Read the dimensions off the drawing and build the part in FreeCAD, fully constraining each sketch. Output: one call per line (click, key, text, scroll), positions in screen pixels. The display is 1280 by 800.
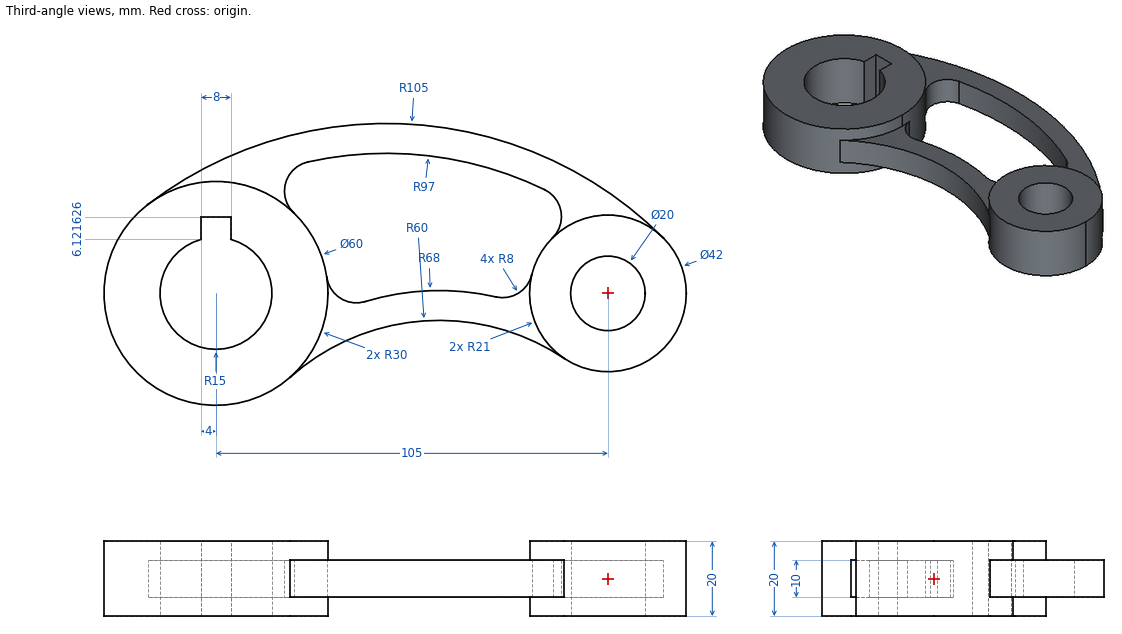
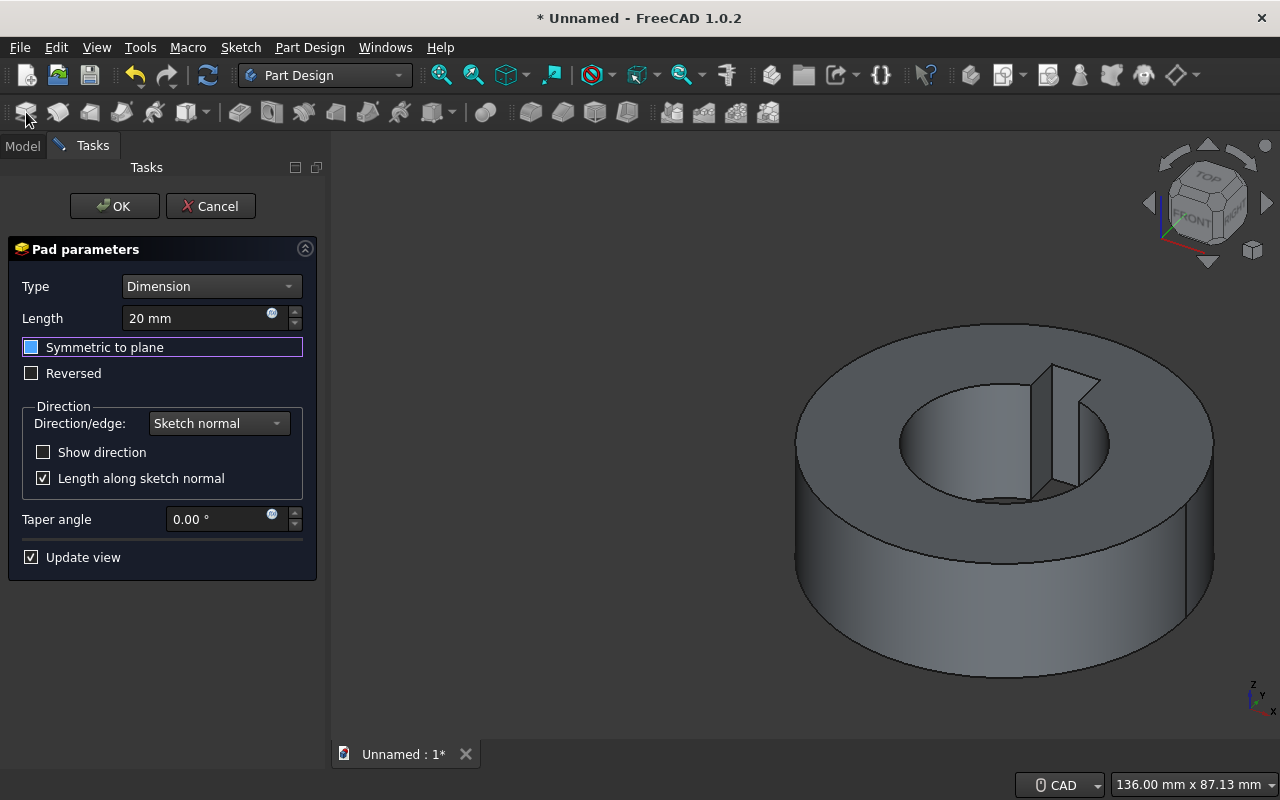
click(30, 347)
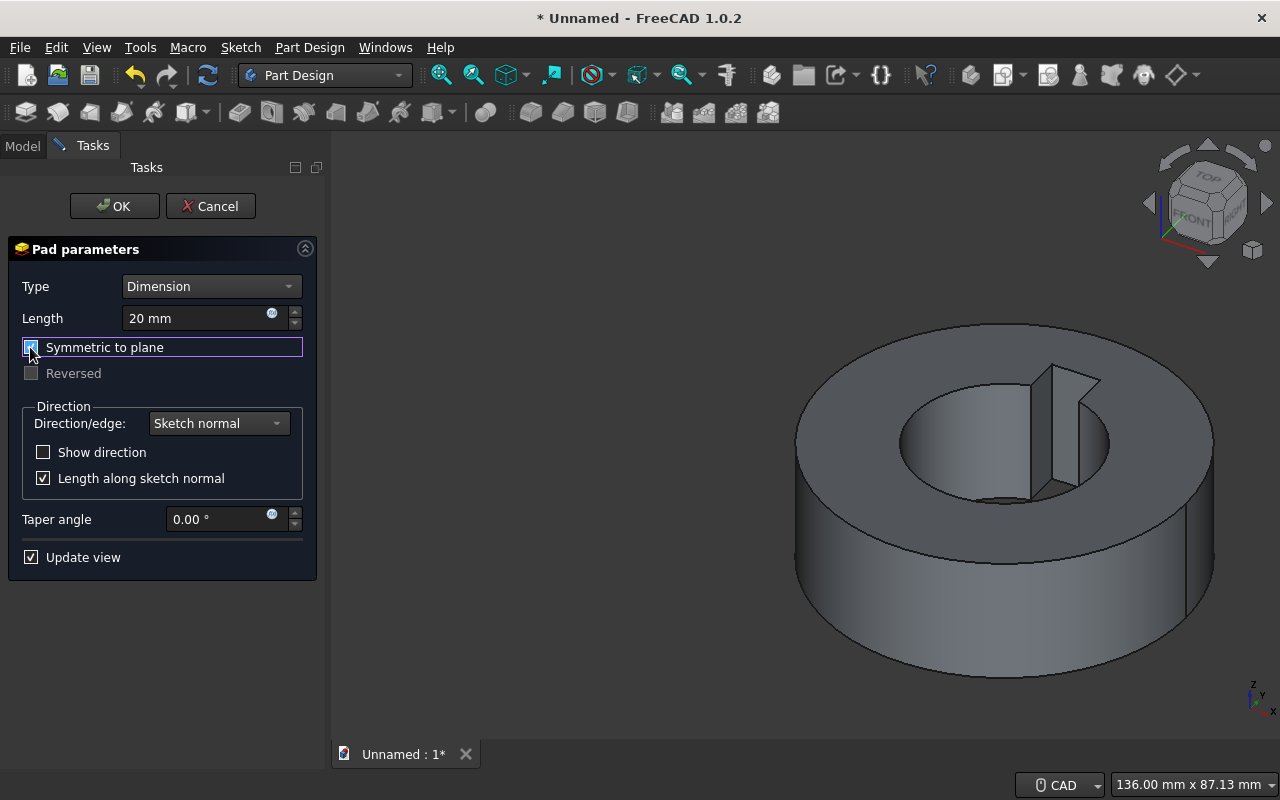
click(115, 206)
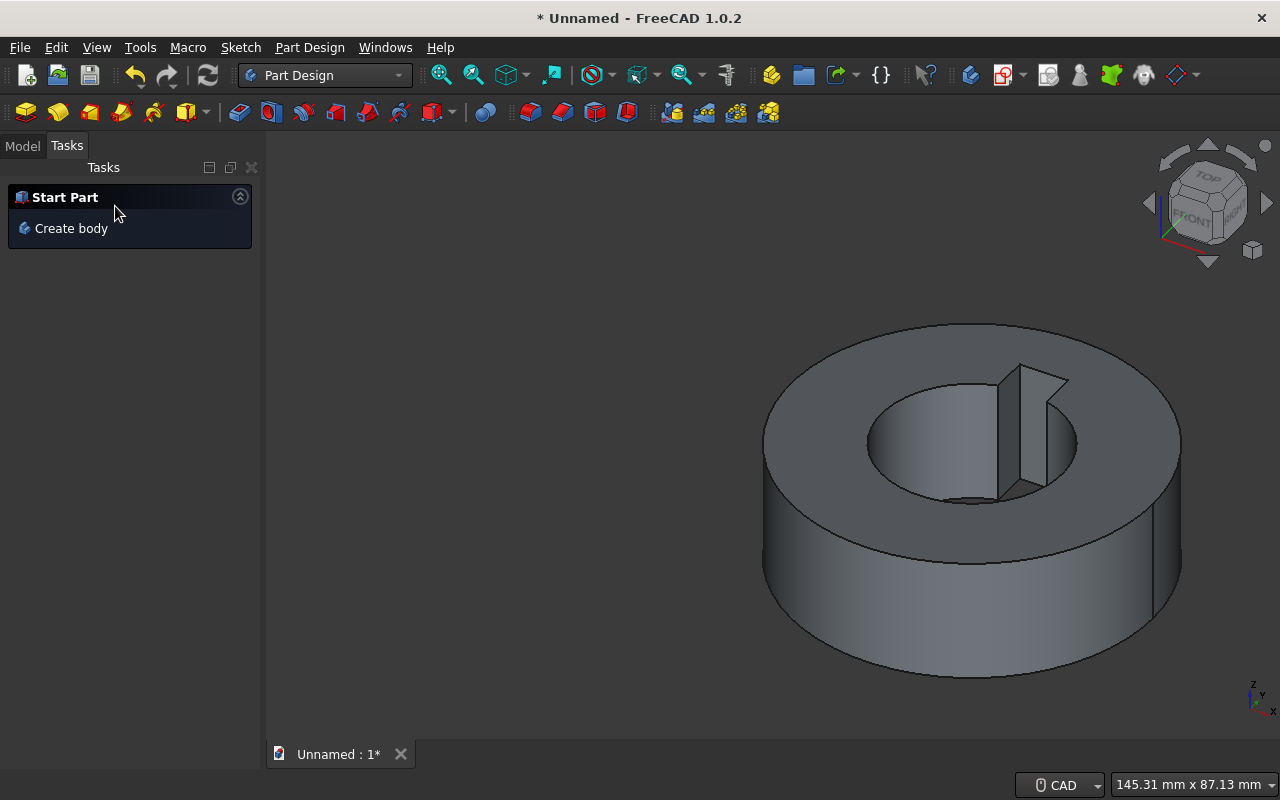
click(442, 76)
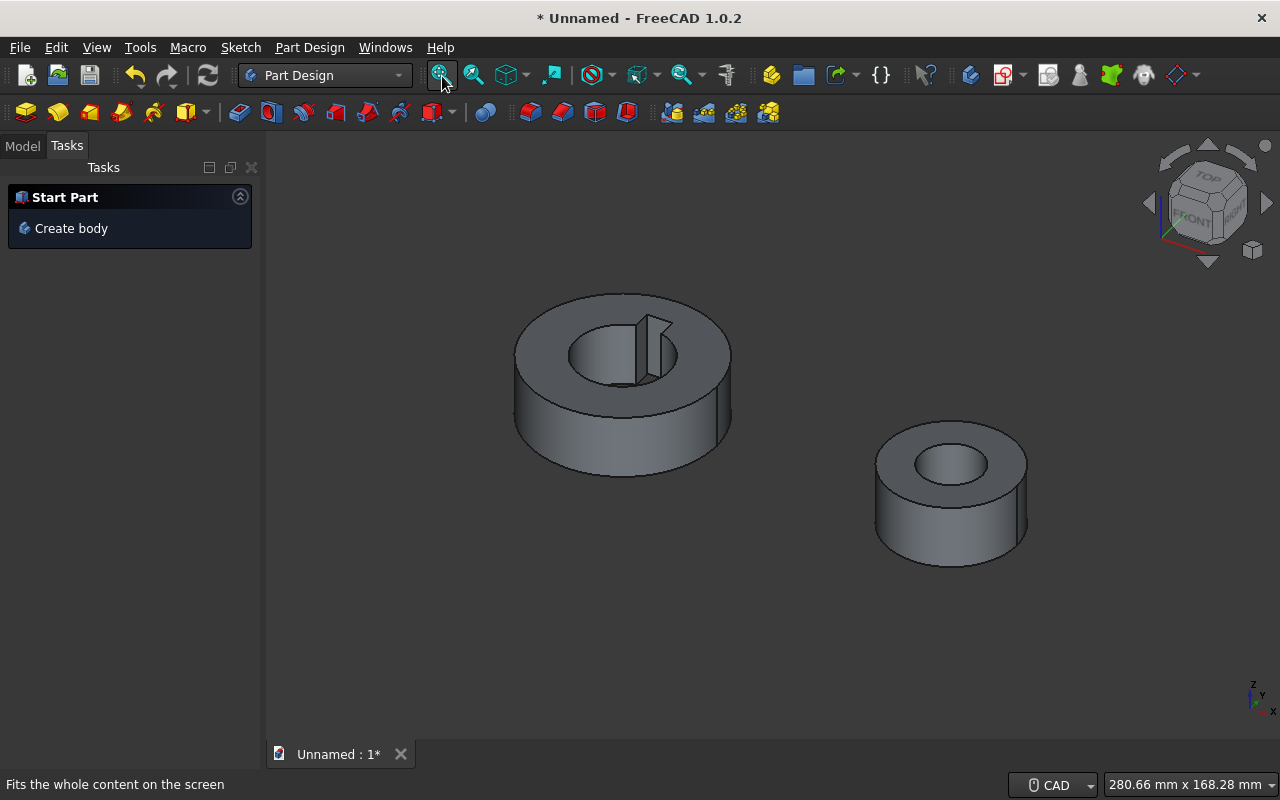
click(23, 145)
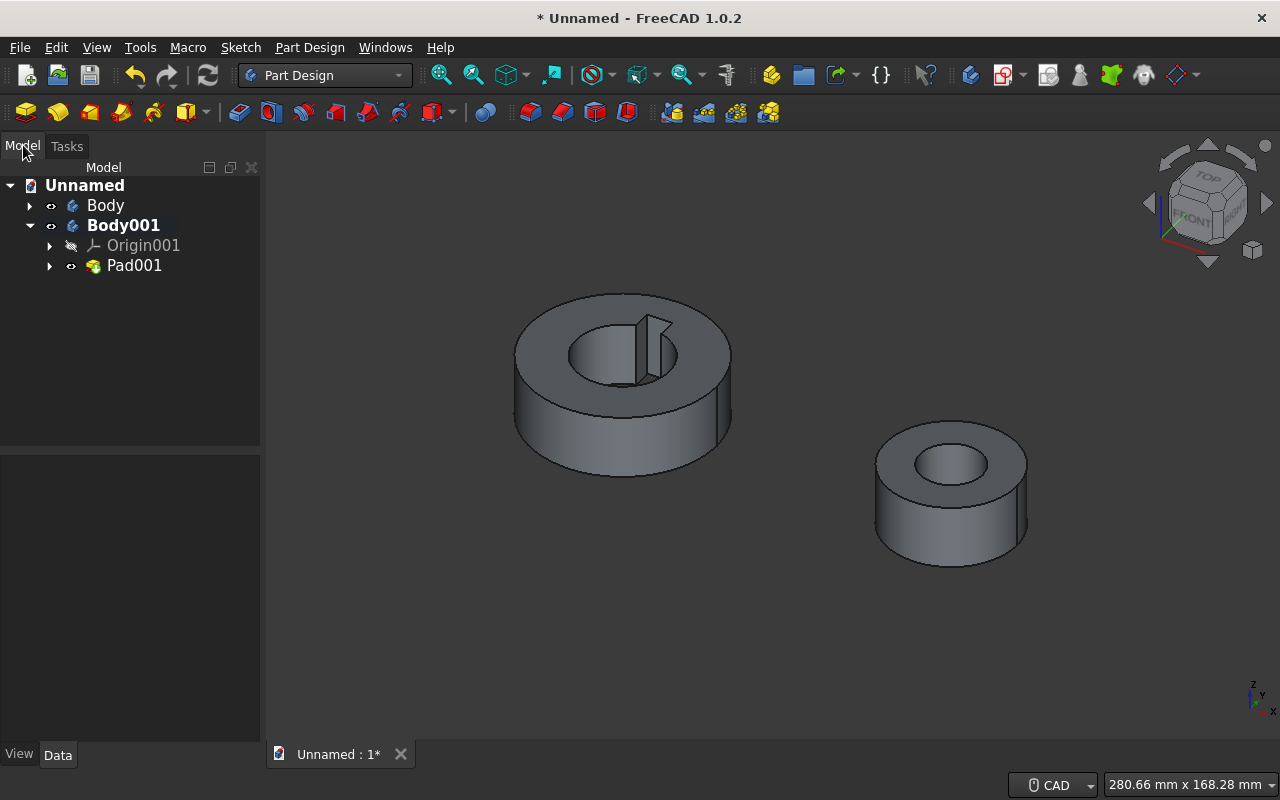
double_click(96, 206)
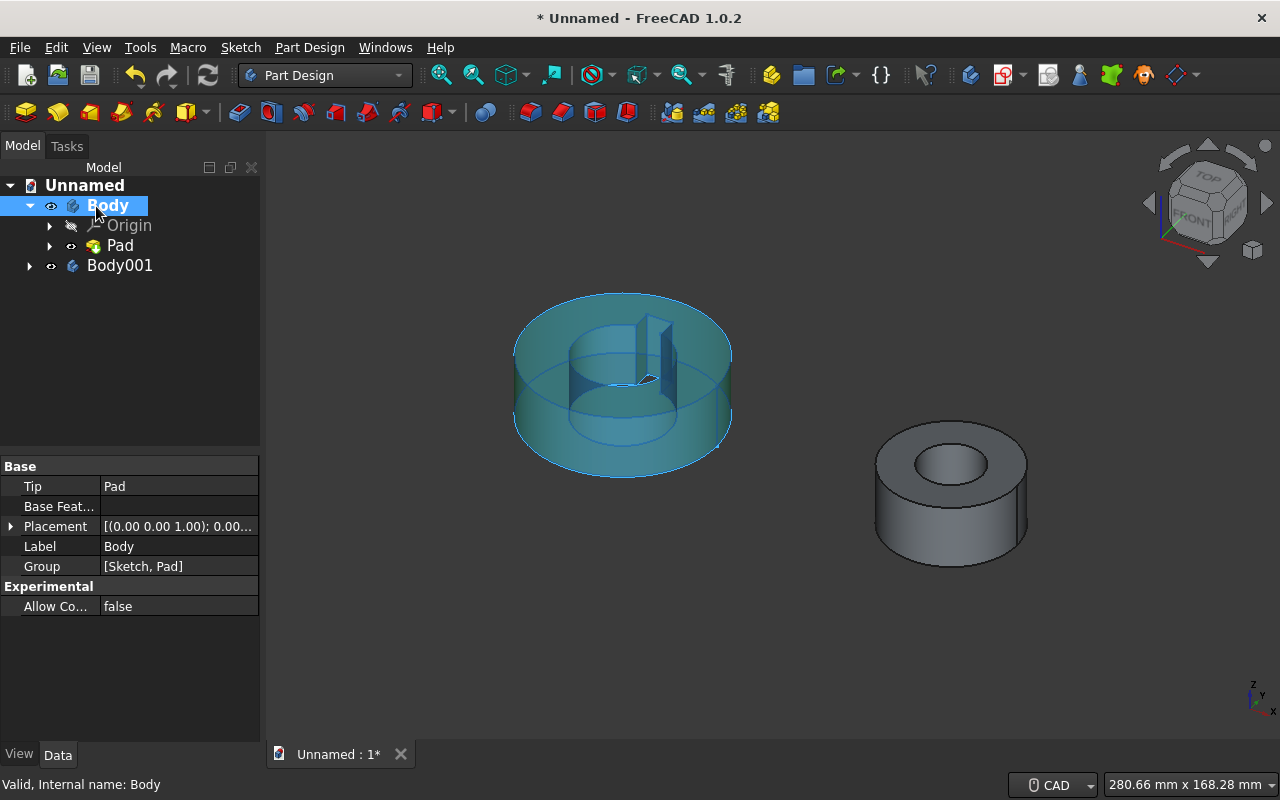
click(96, 206)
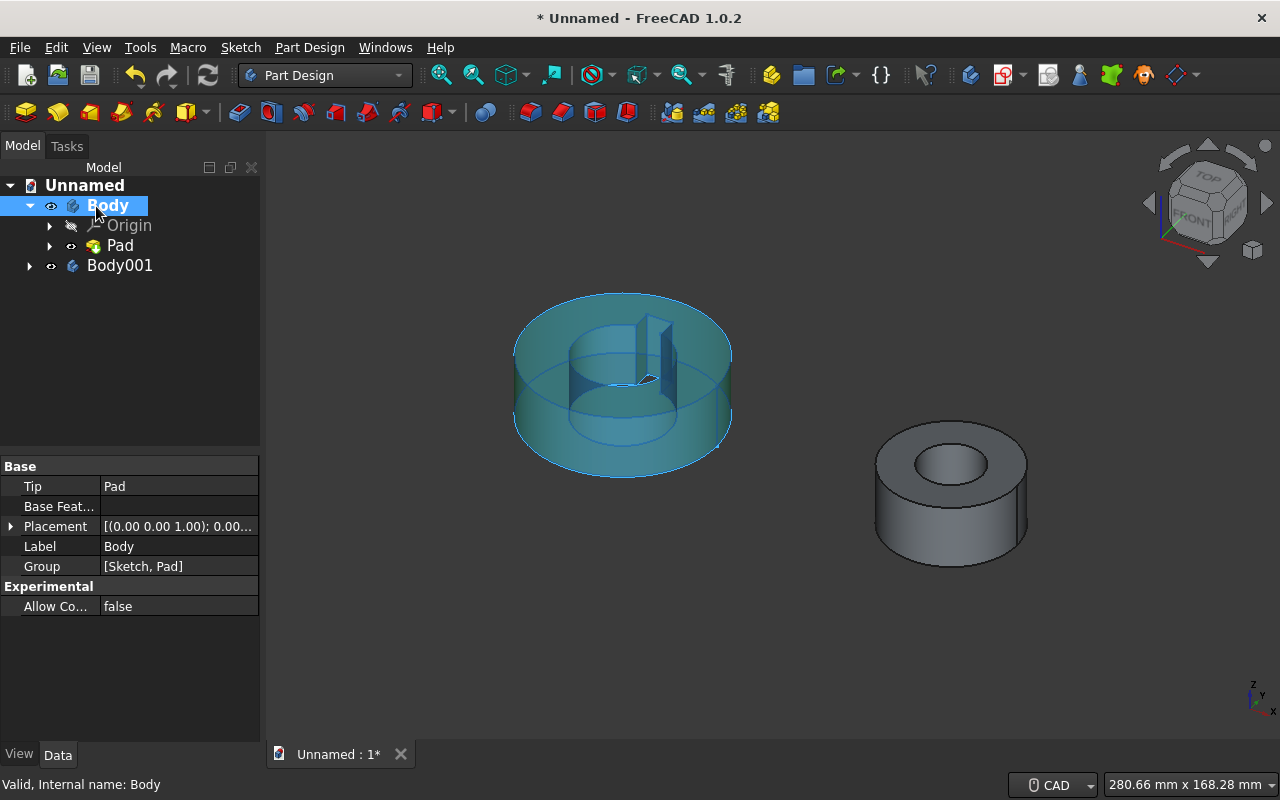
click(146, 606)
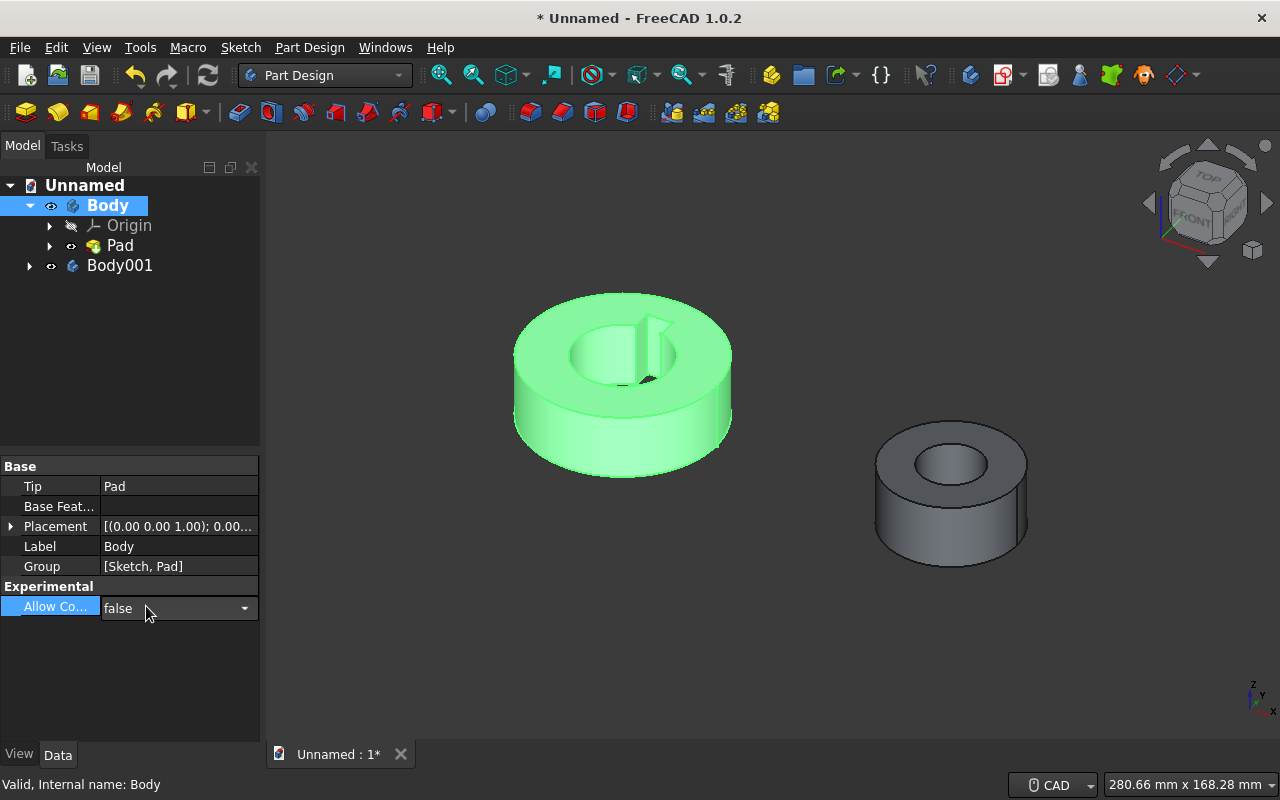
click(146, 606)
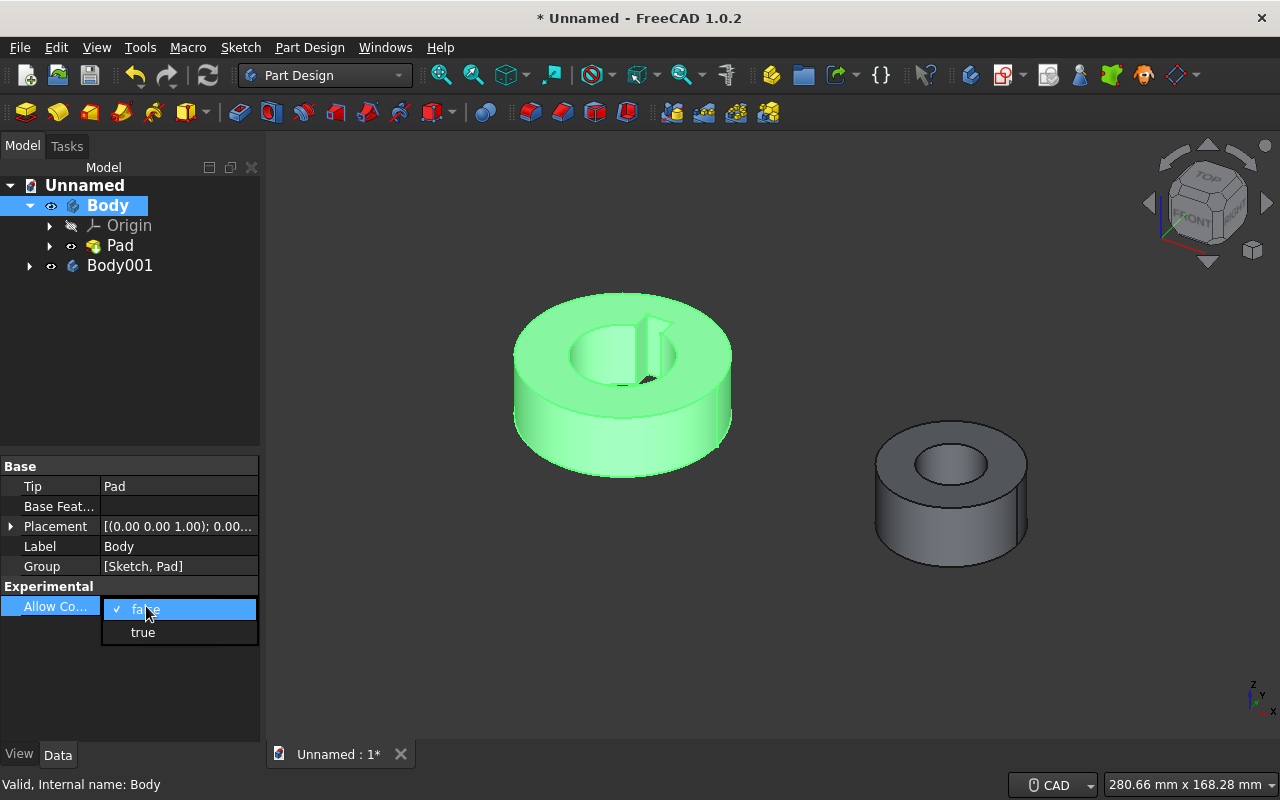
click(179, 632)
key(Return)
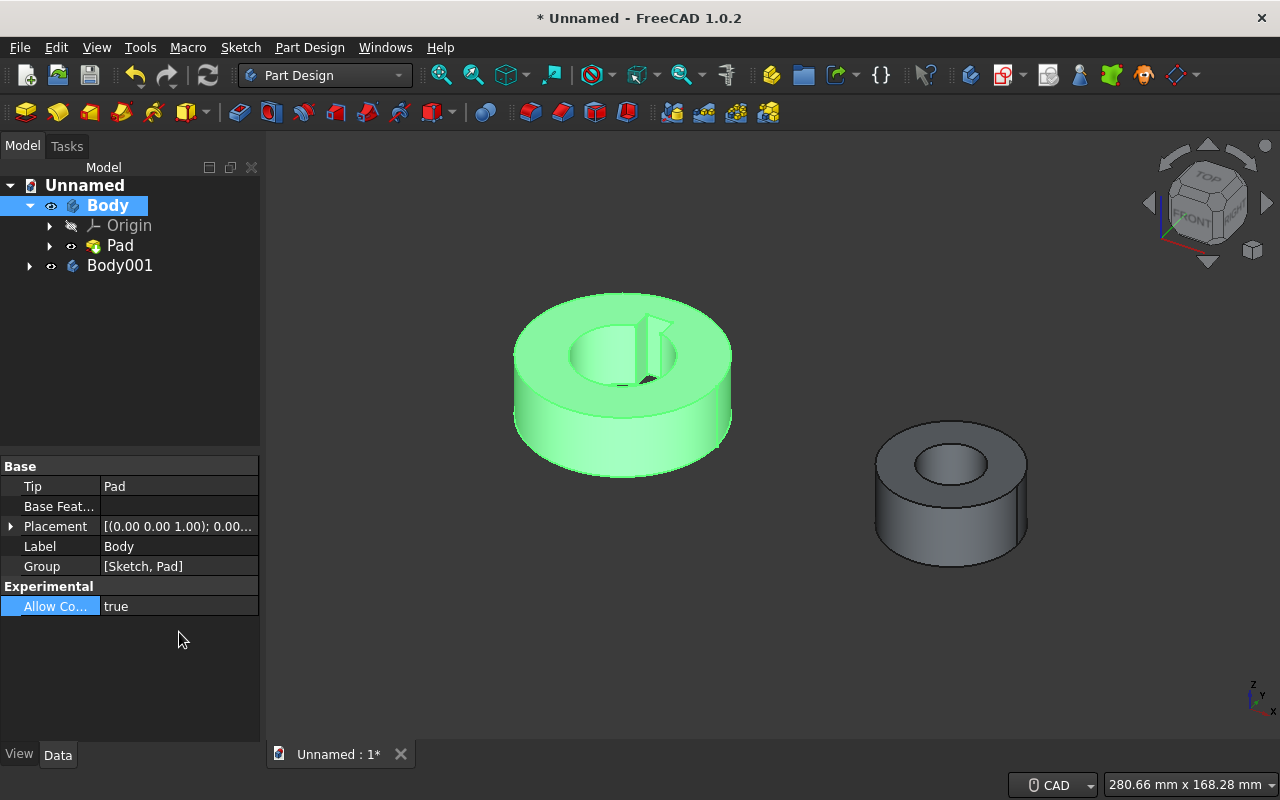
click(96, 266)